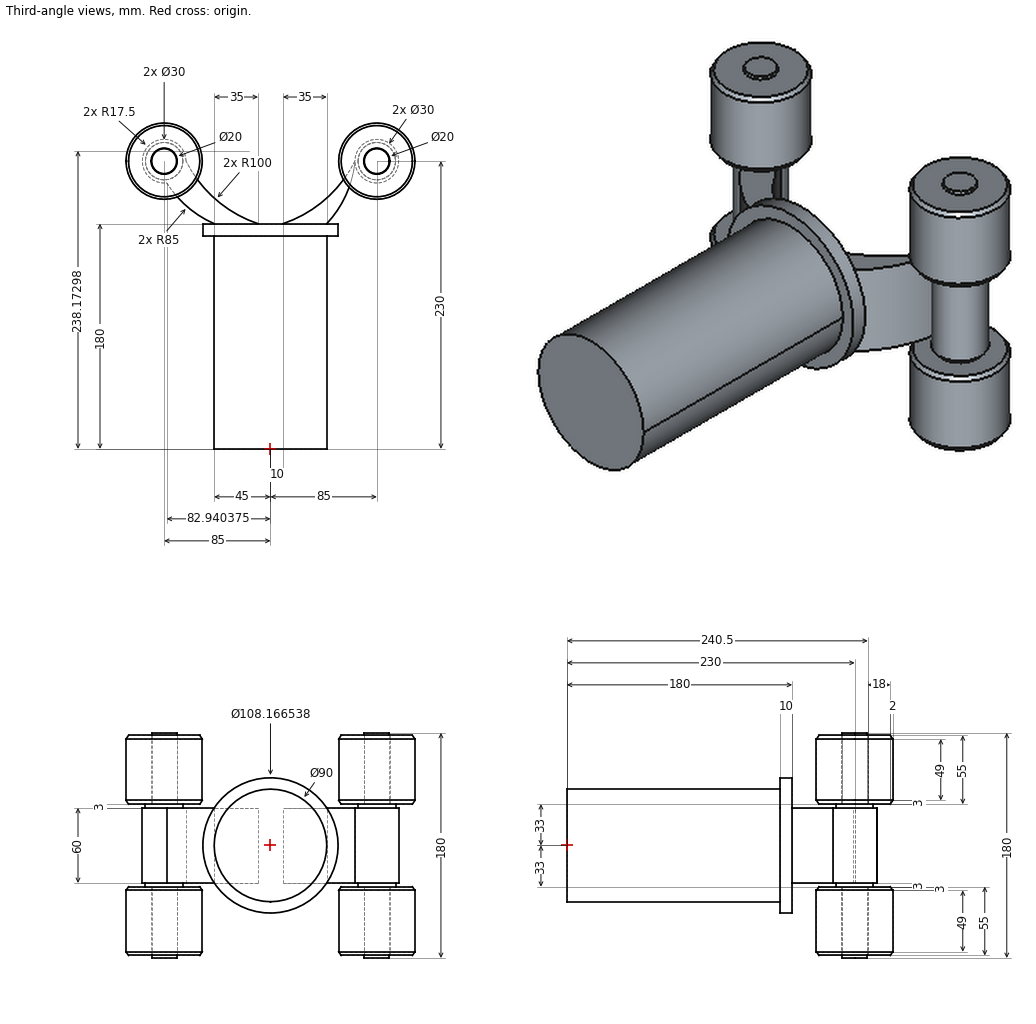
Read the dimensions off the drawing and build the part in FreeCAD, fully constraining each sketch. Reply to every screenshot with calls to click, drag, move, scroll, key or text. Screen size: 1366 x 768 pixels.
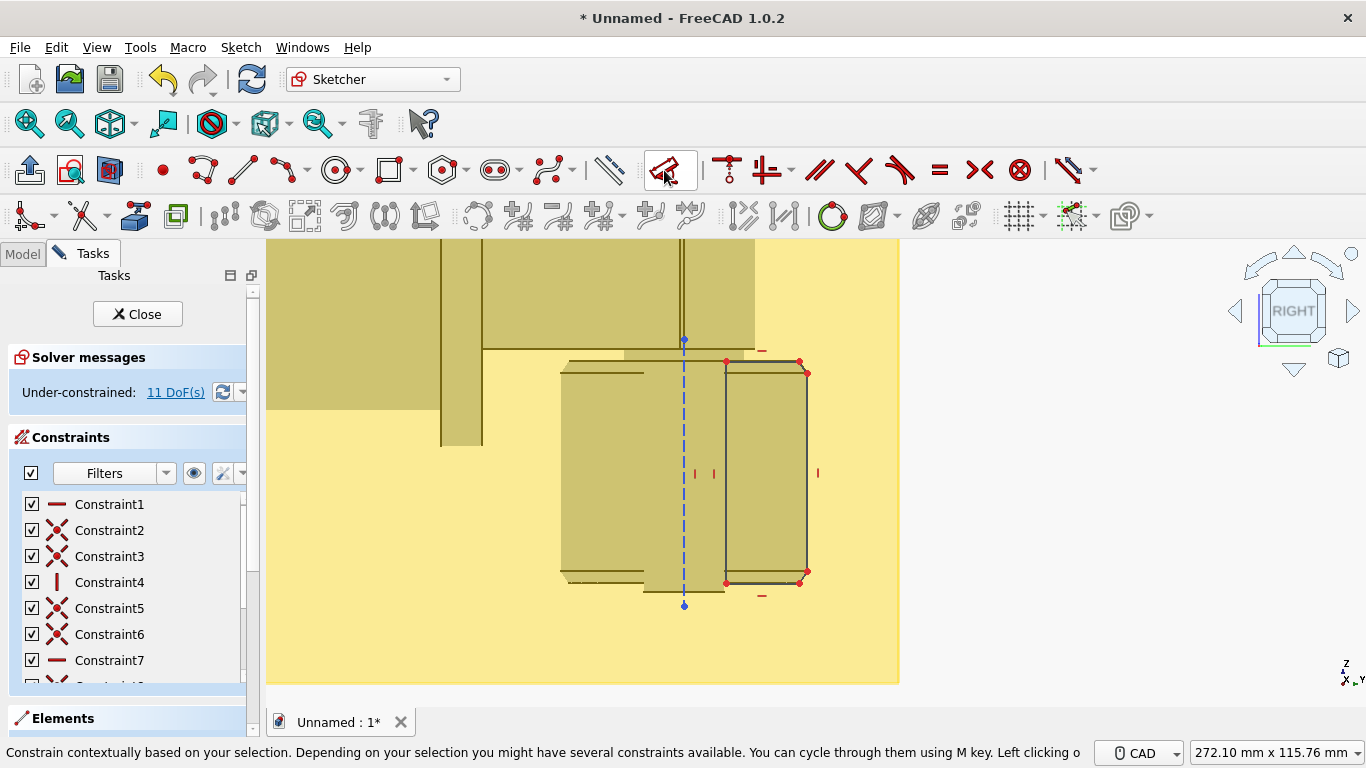
click(748, 362)
click(763, 328)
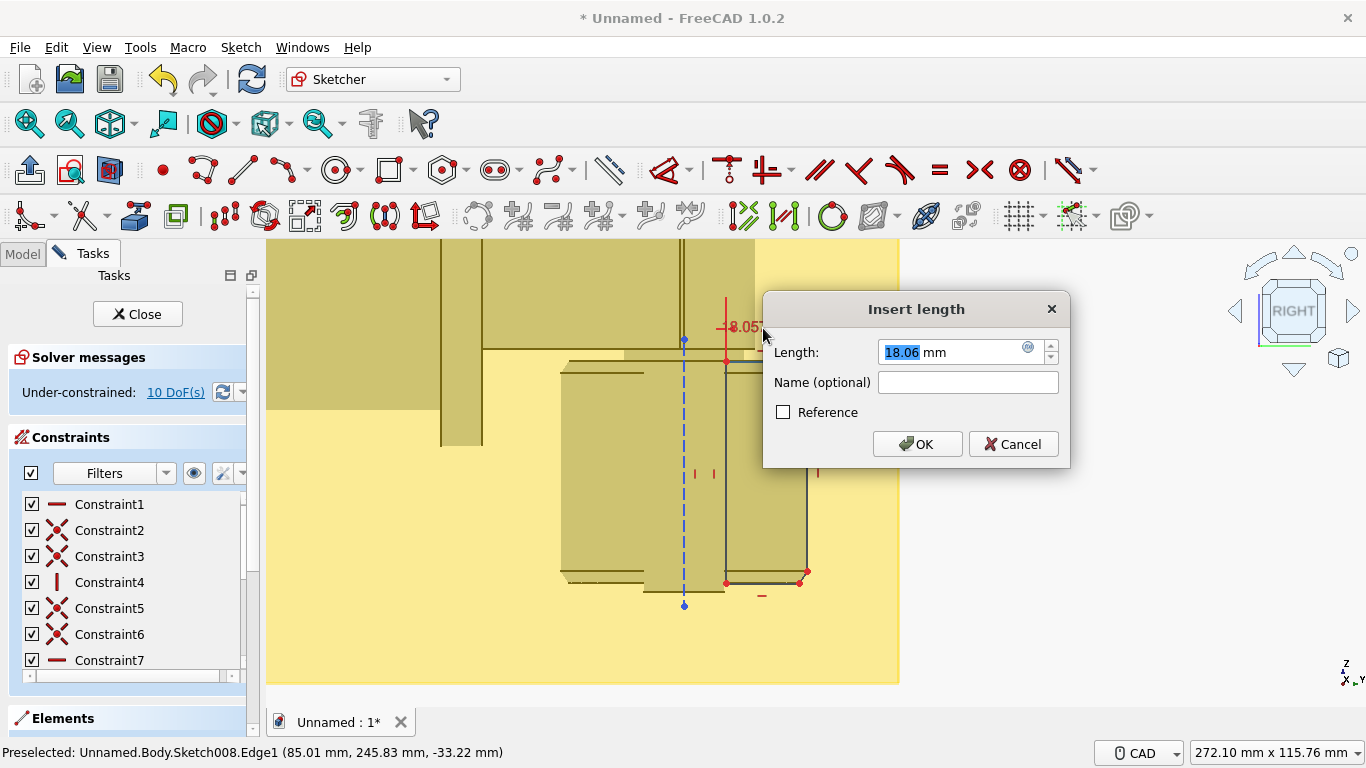
text(18)
key(Return)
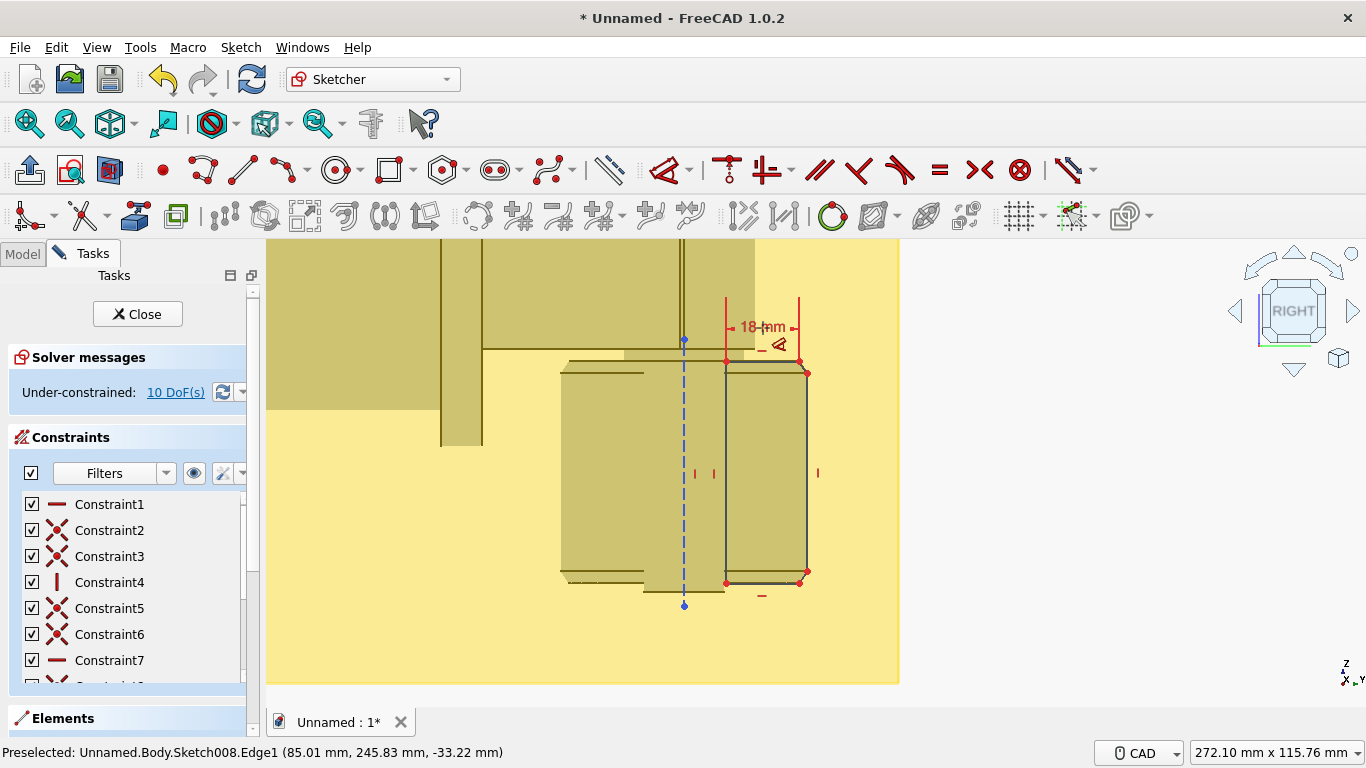
click(807, 433)
click(841, 473)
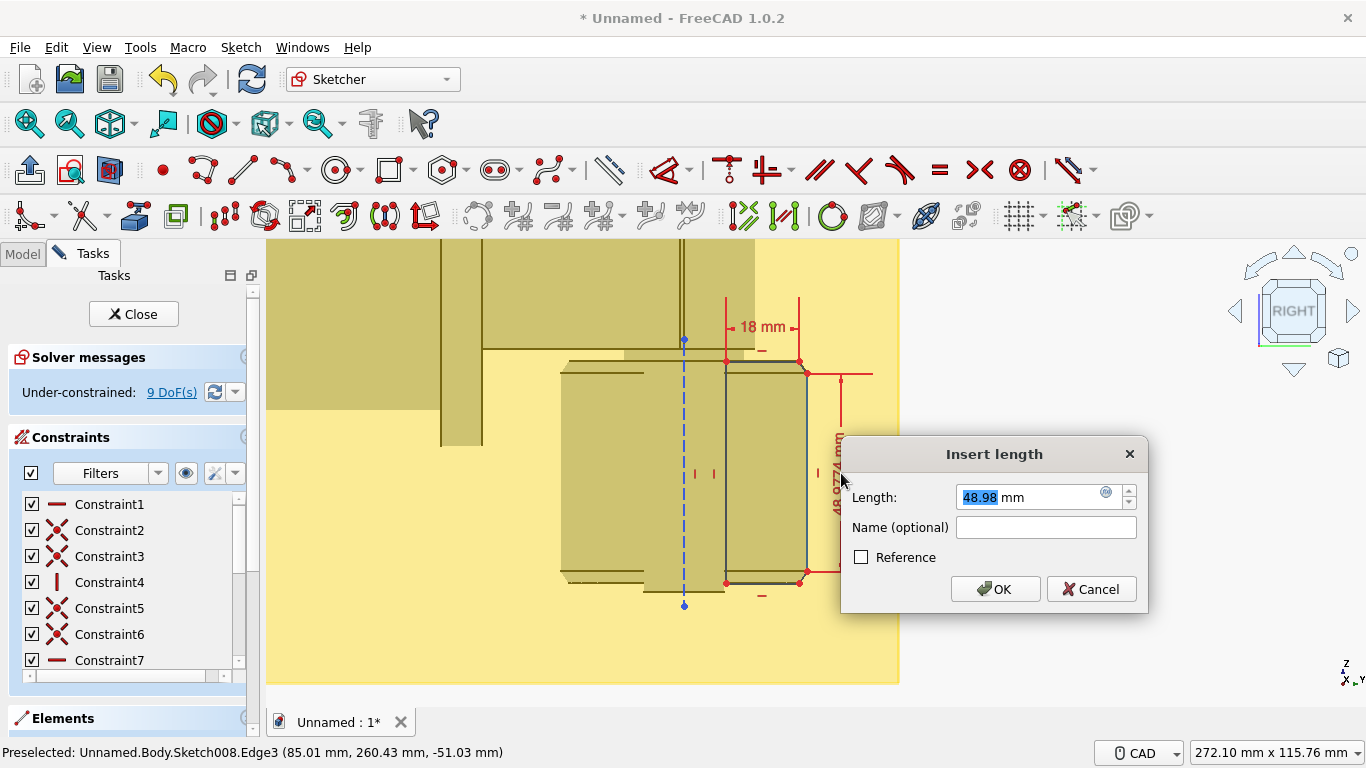
text(49)
key(Return)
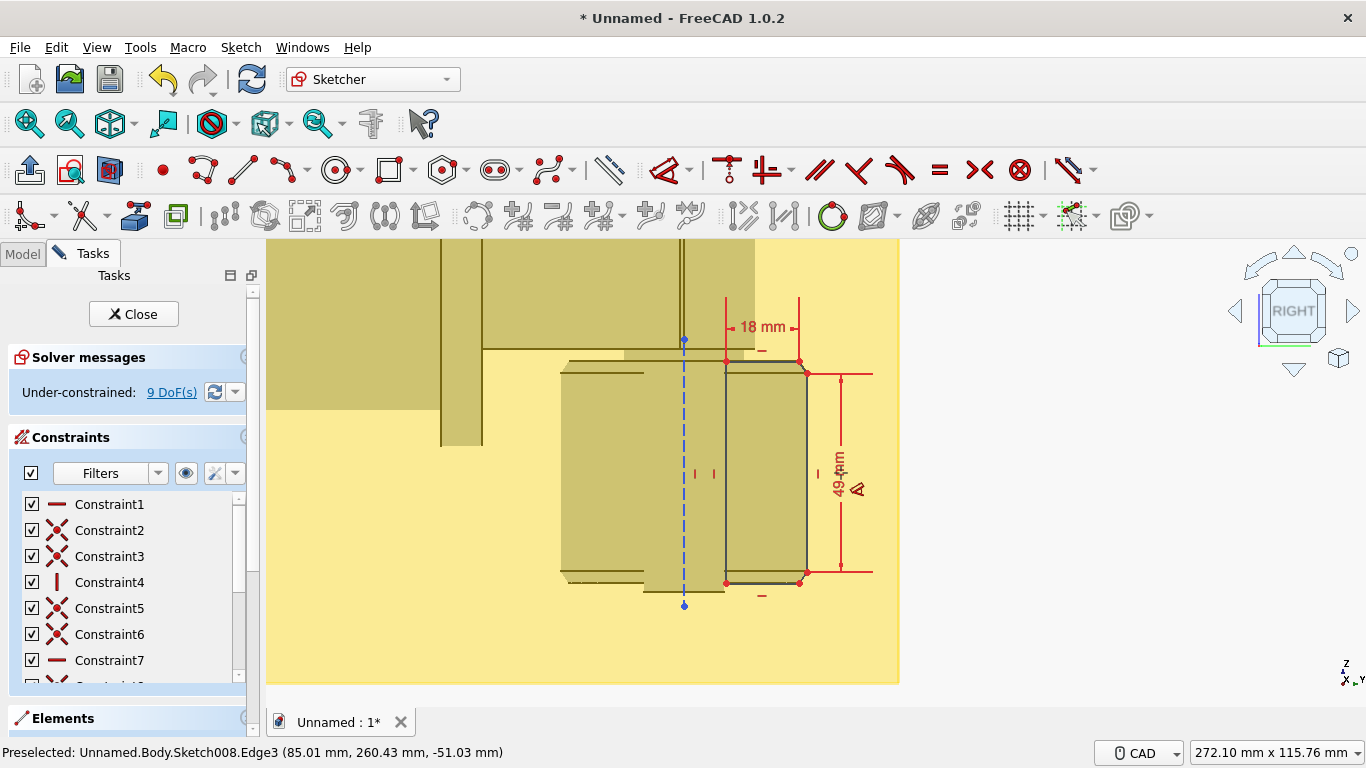
click(777, 584)
click(763, 618)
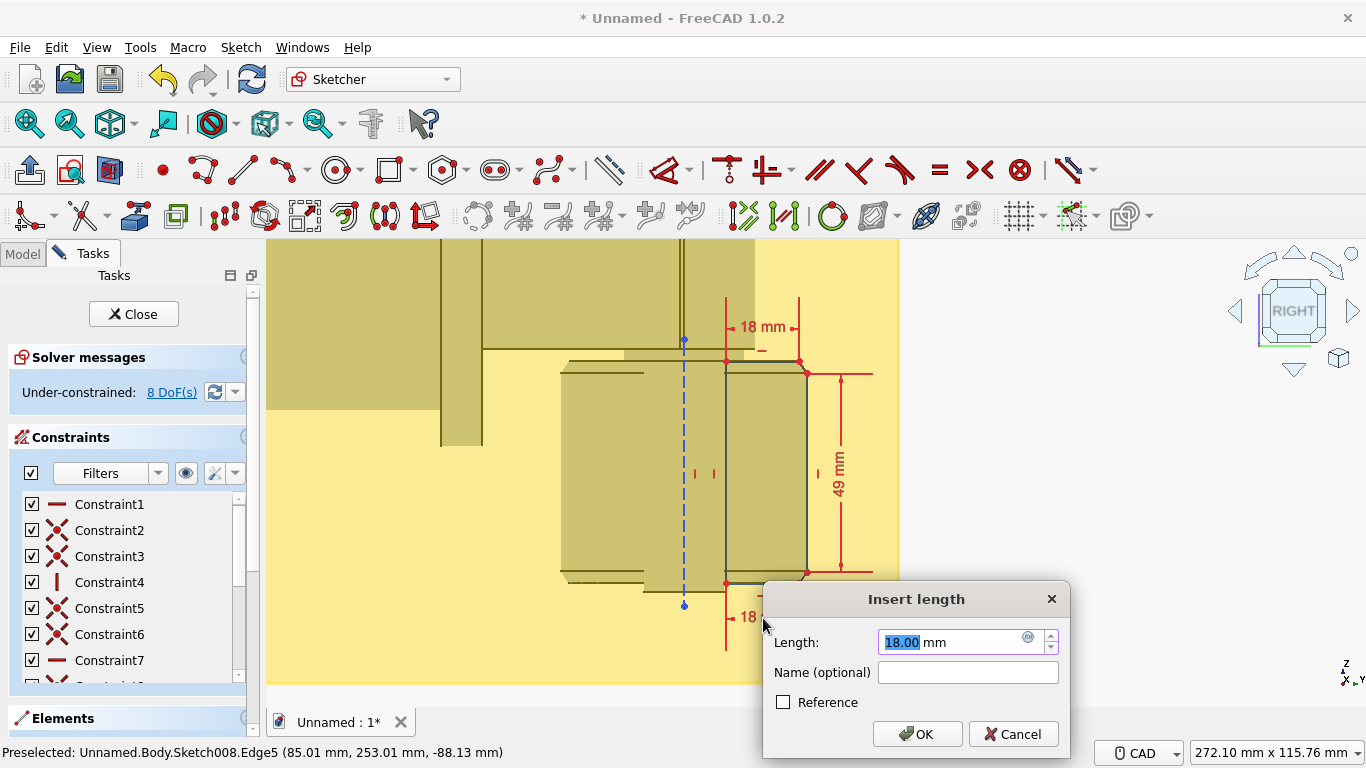
text(18)
key(Return)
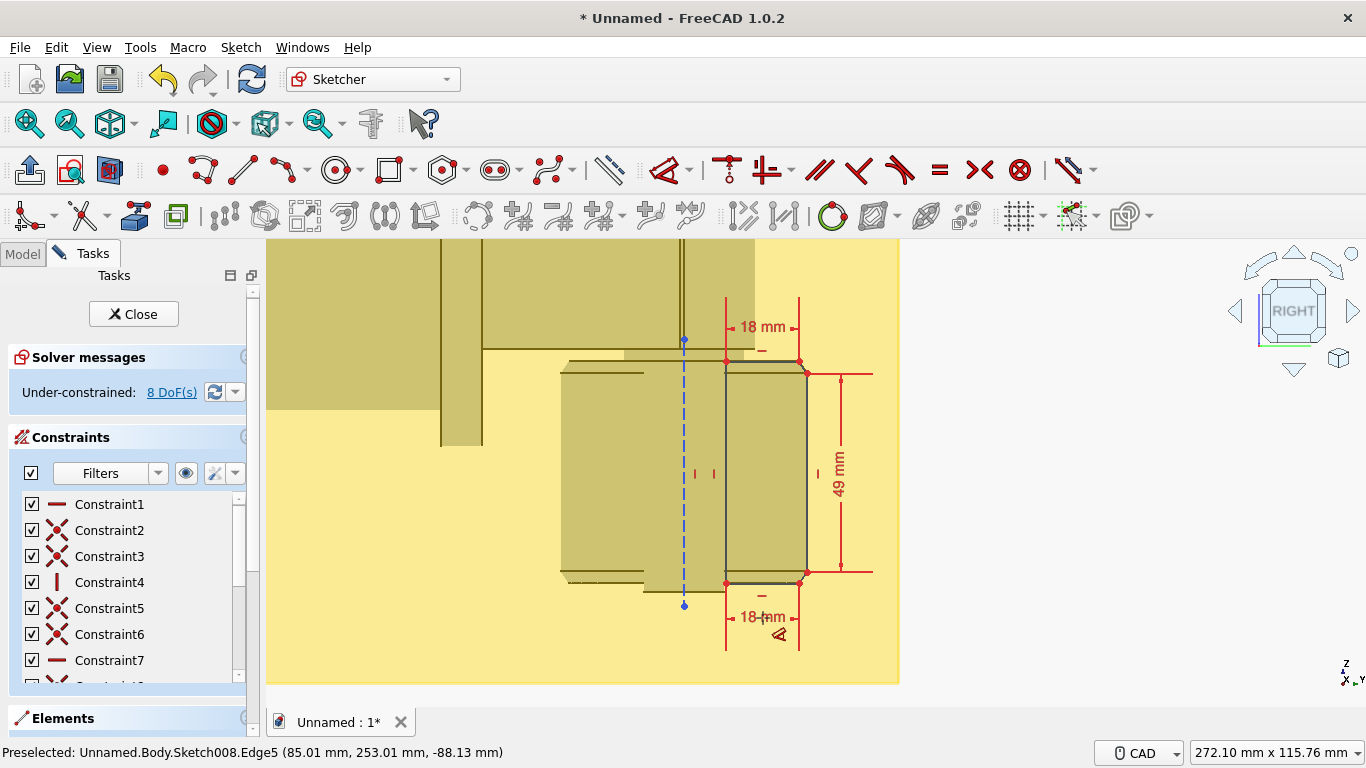
click(726, 517)
click(760, 473)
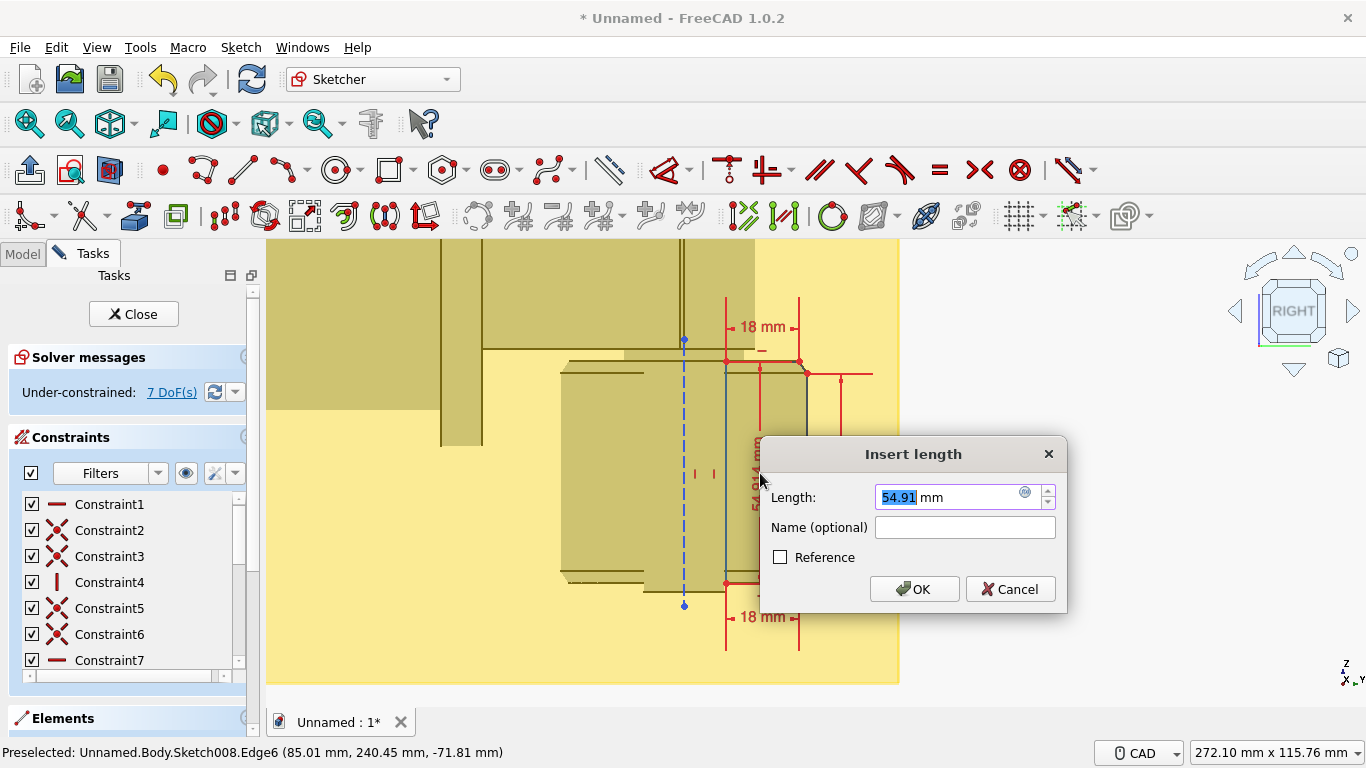
text(55)
key(Return)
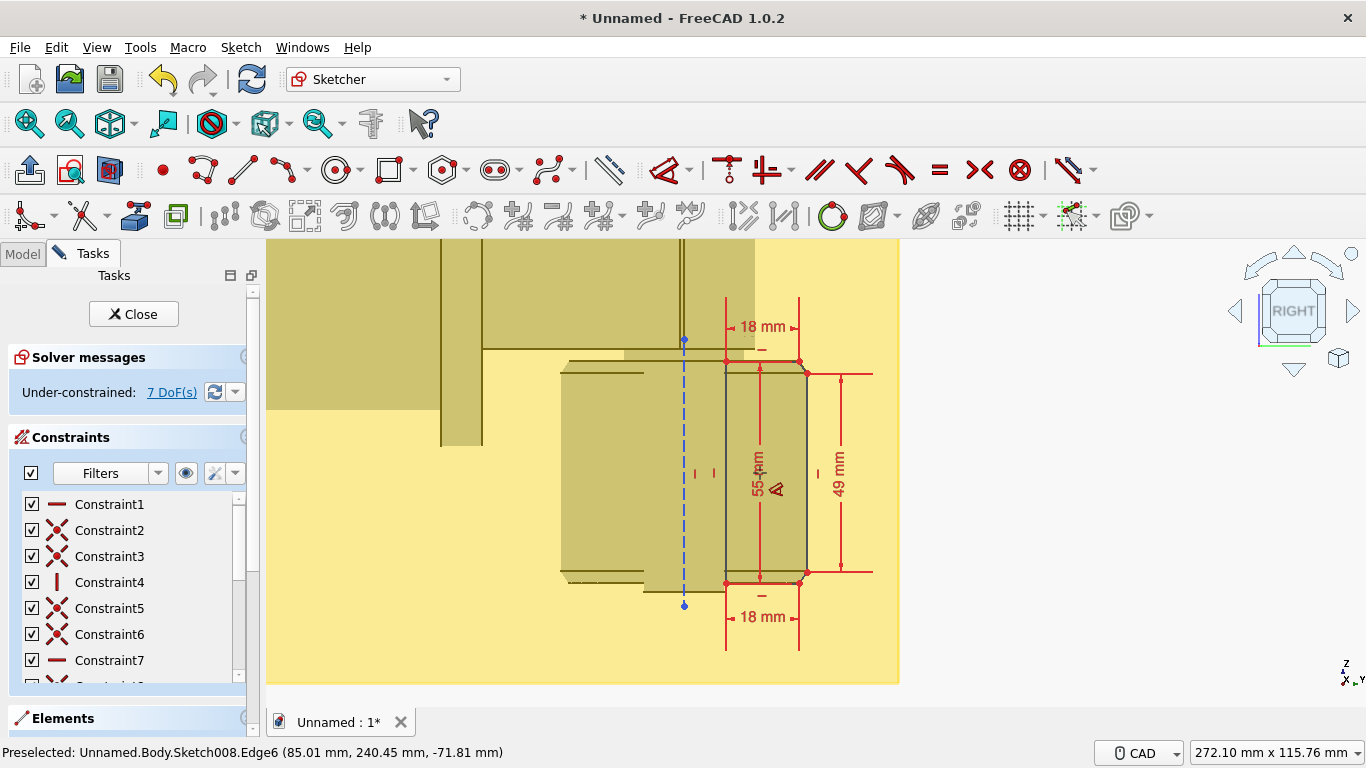
scroll(803, 368, up, 8)